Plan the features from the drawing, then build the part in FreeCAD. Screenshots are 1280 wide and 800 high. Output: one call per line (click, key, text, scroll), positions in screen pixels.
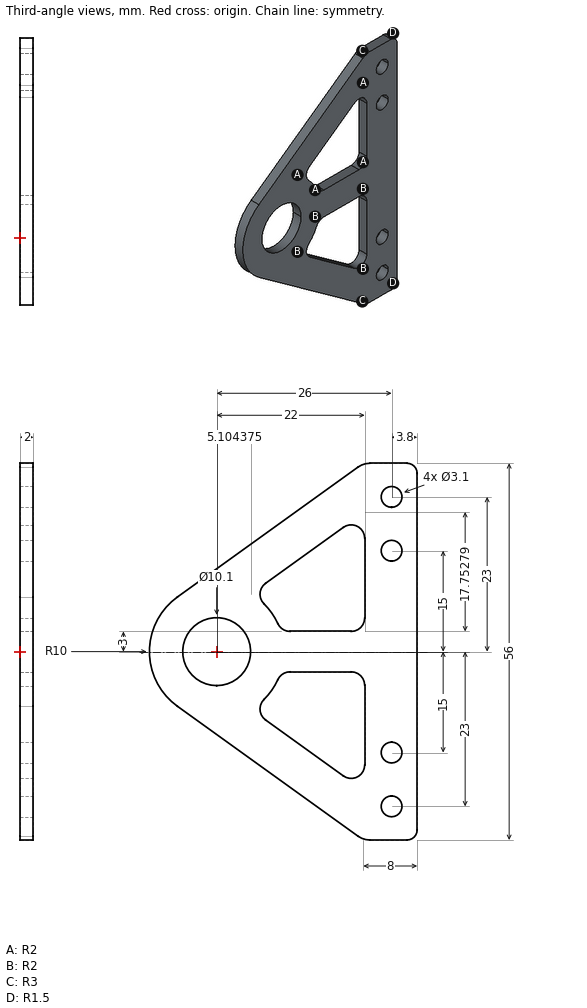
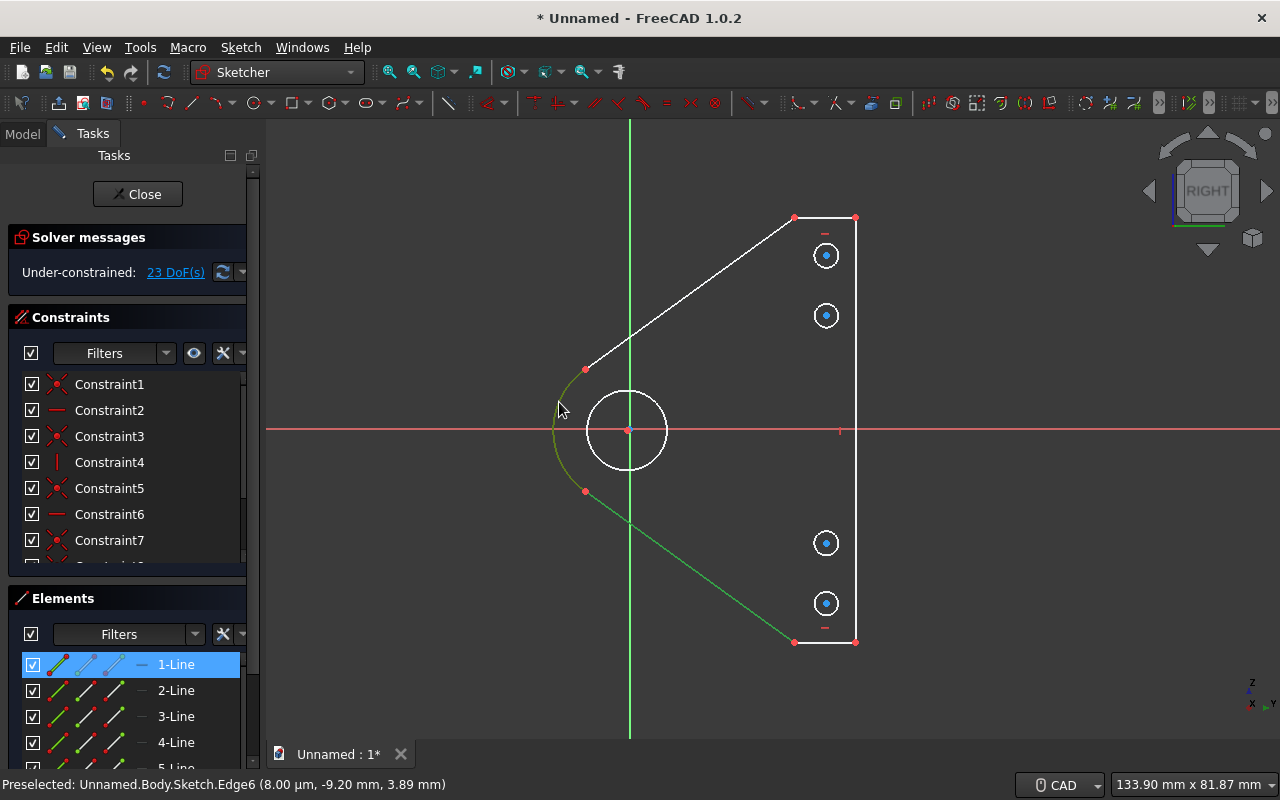
click(644, 104)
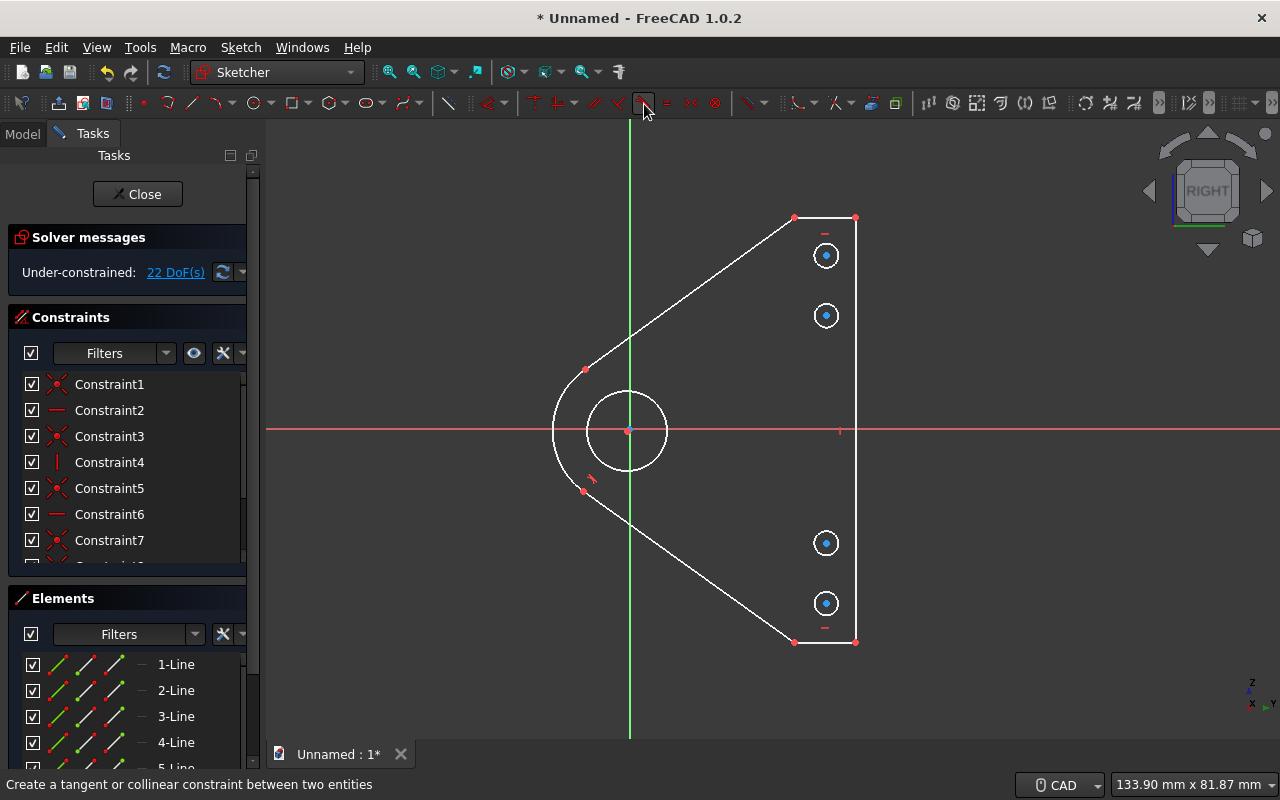
click(732, 263)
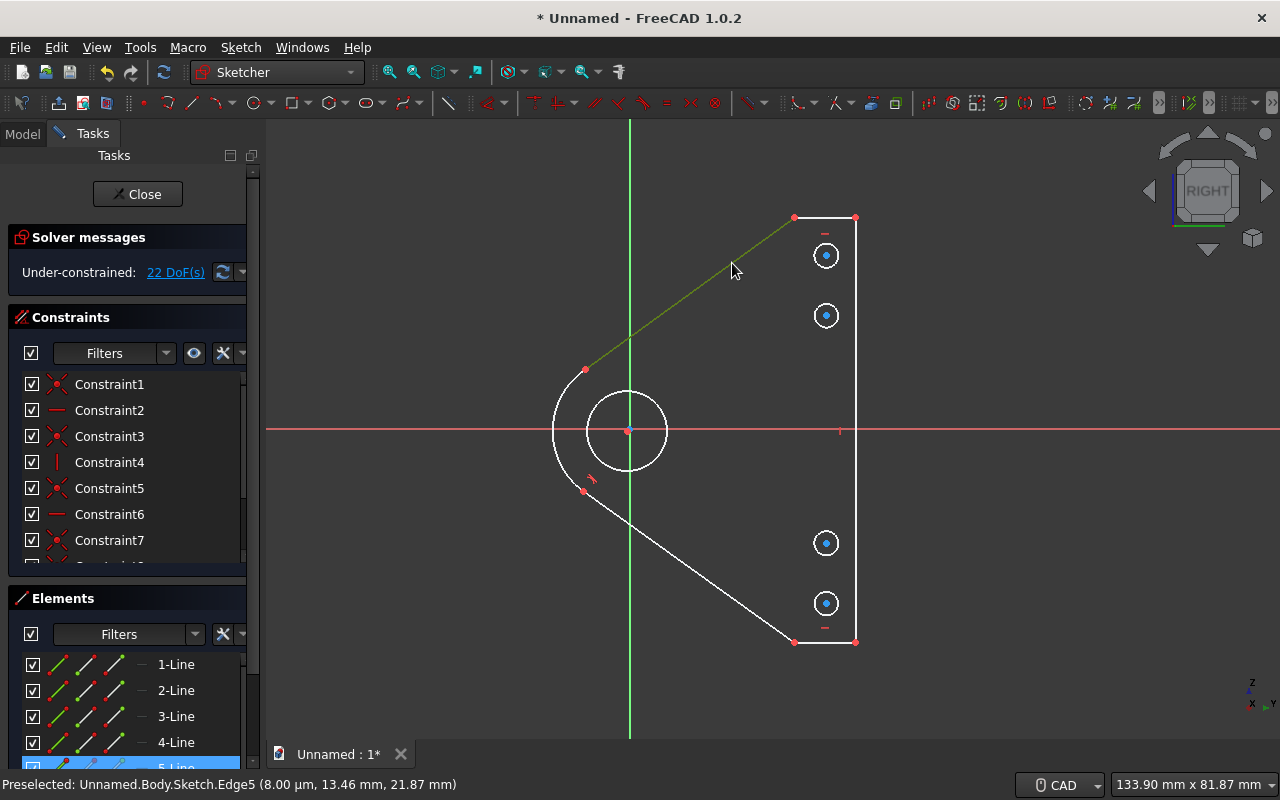
click(559, 402)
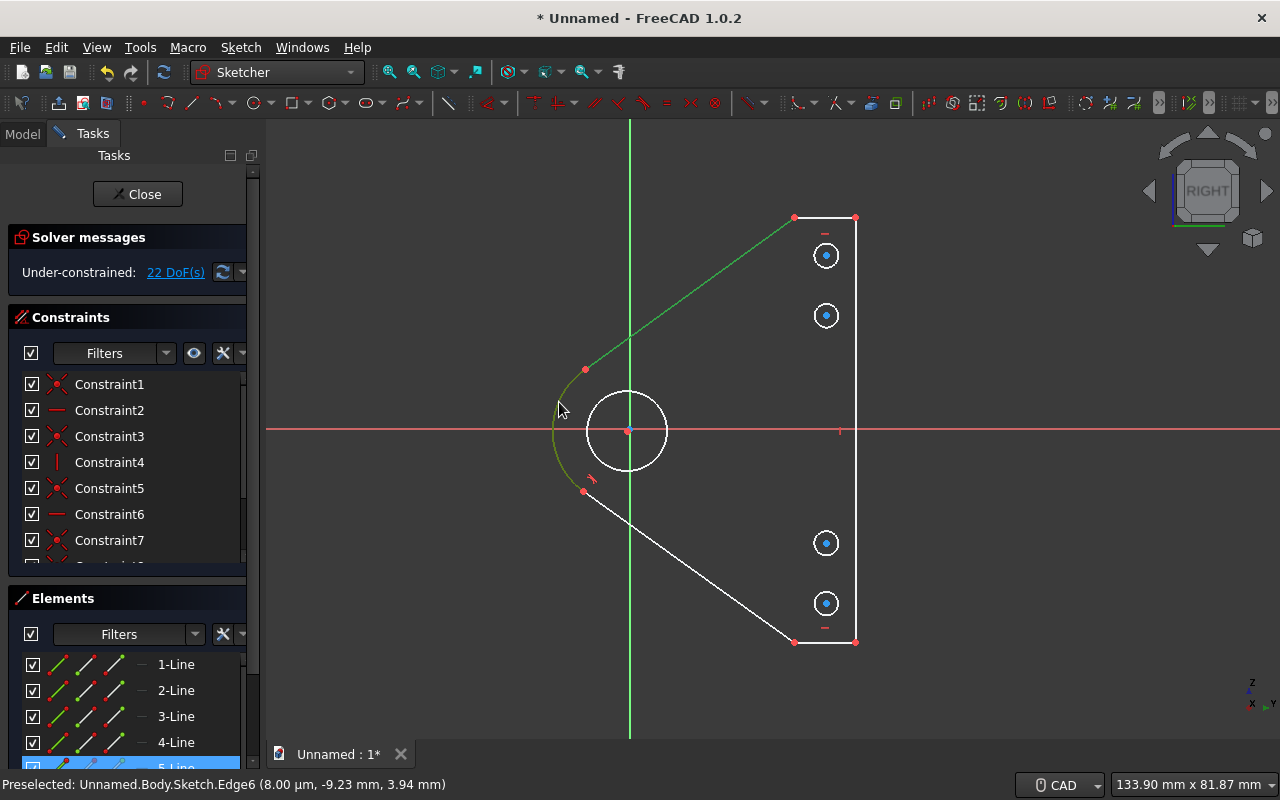
click(644, 104)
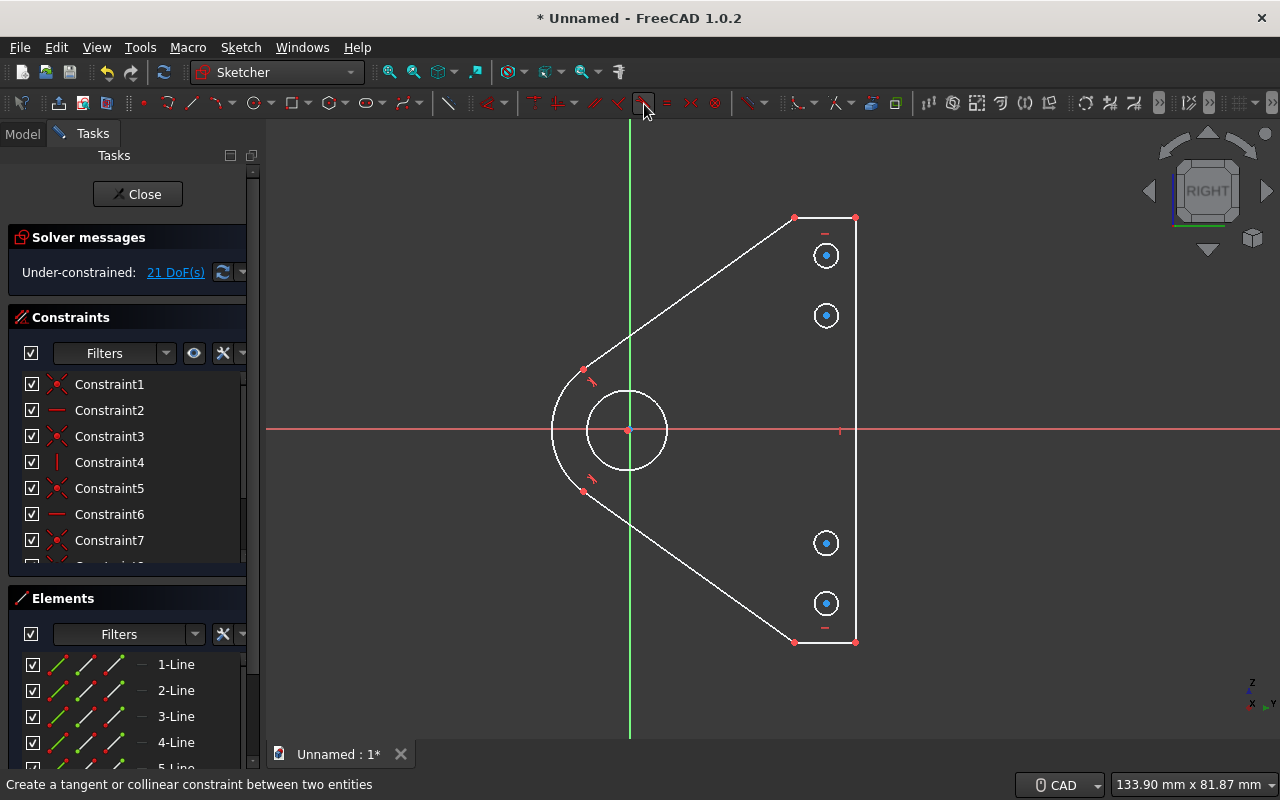
scroll(628, 430, up, 7)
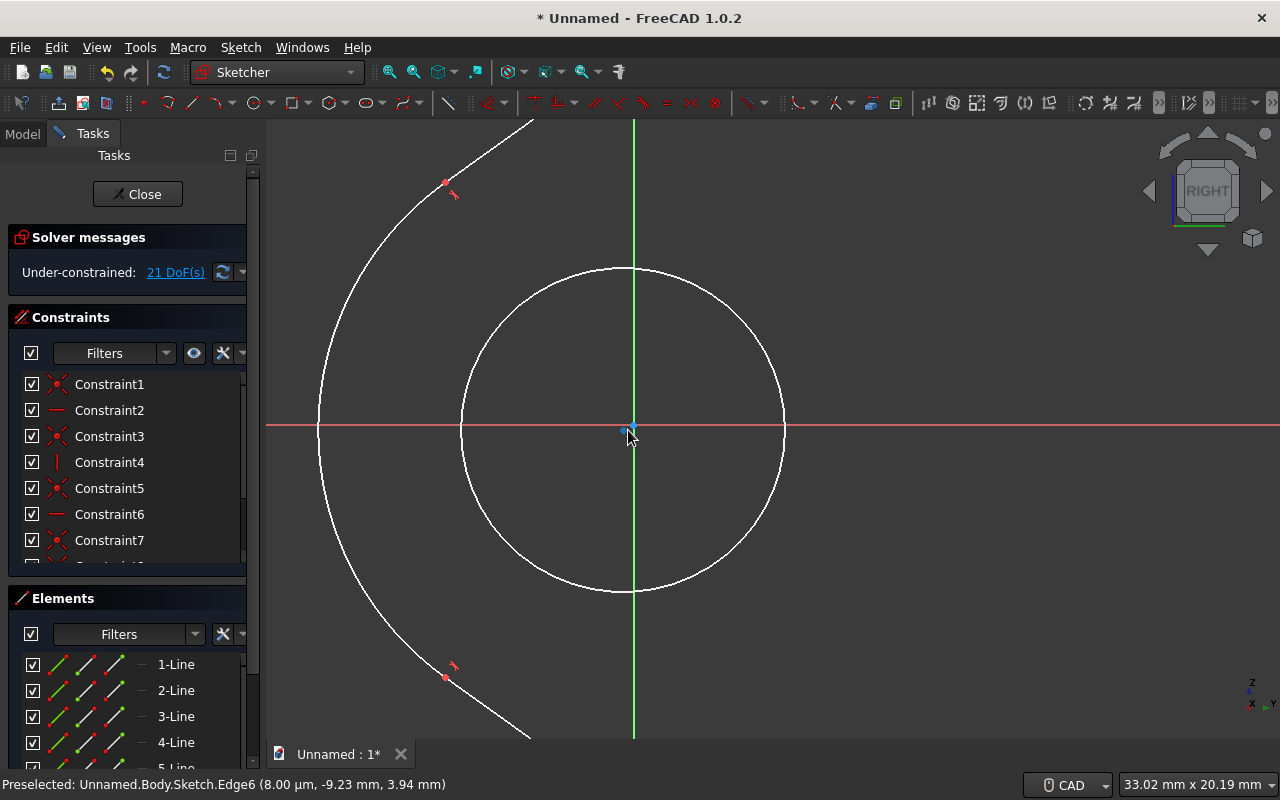
drag(613, 415, 644, 440)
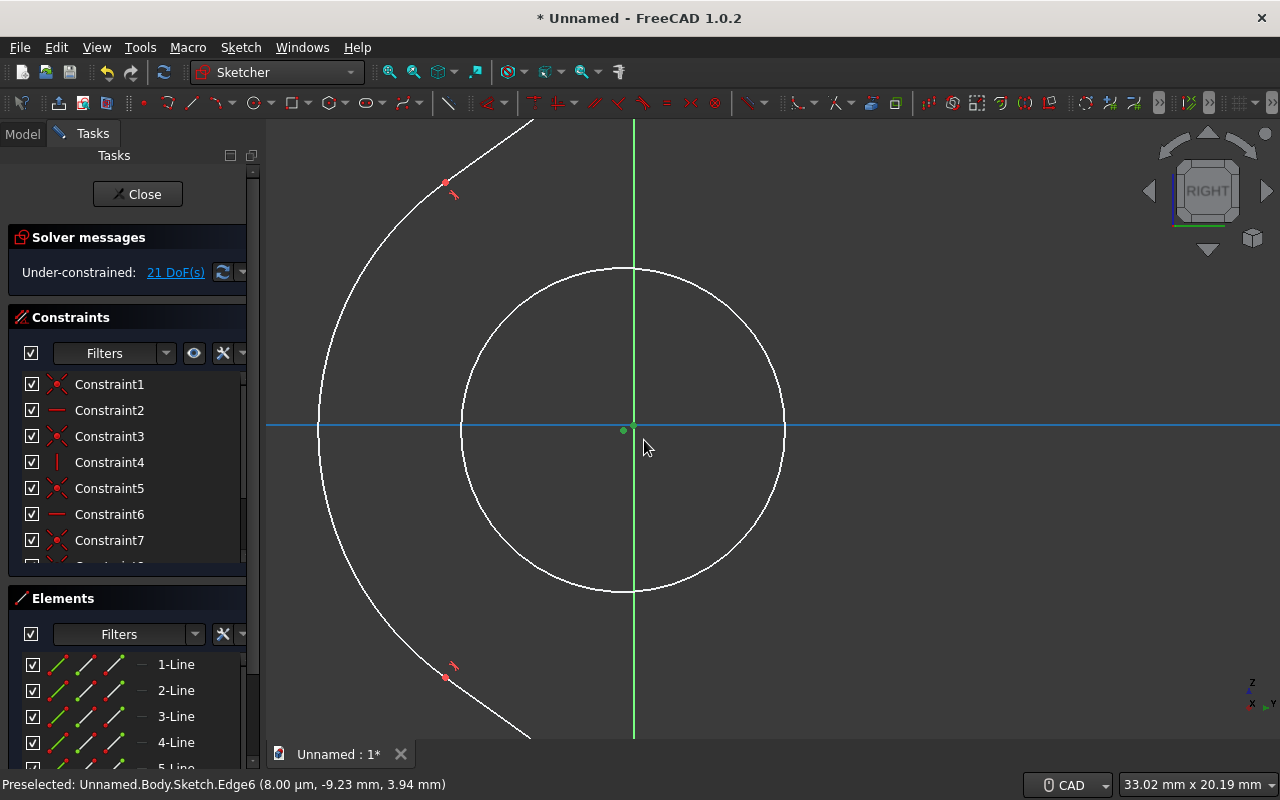
click(534, 104)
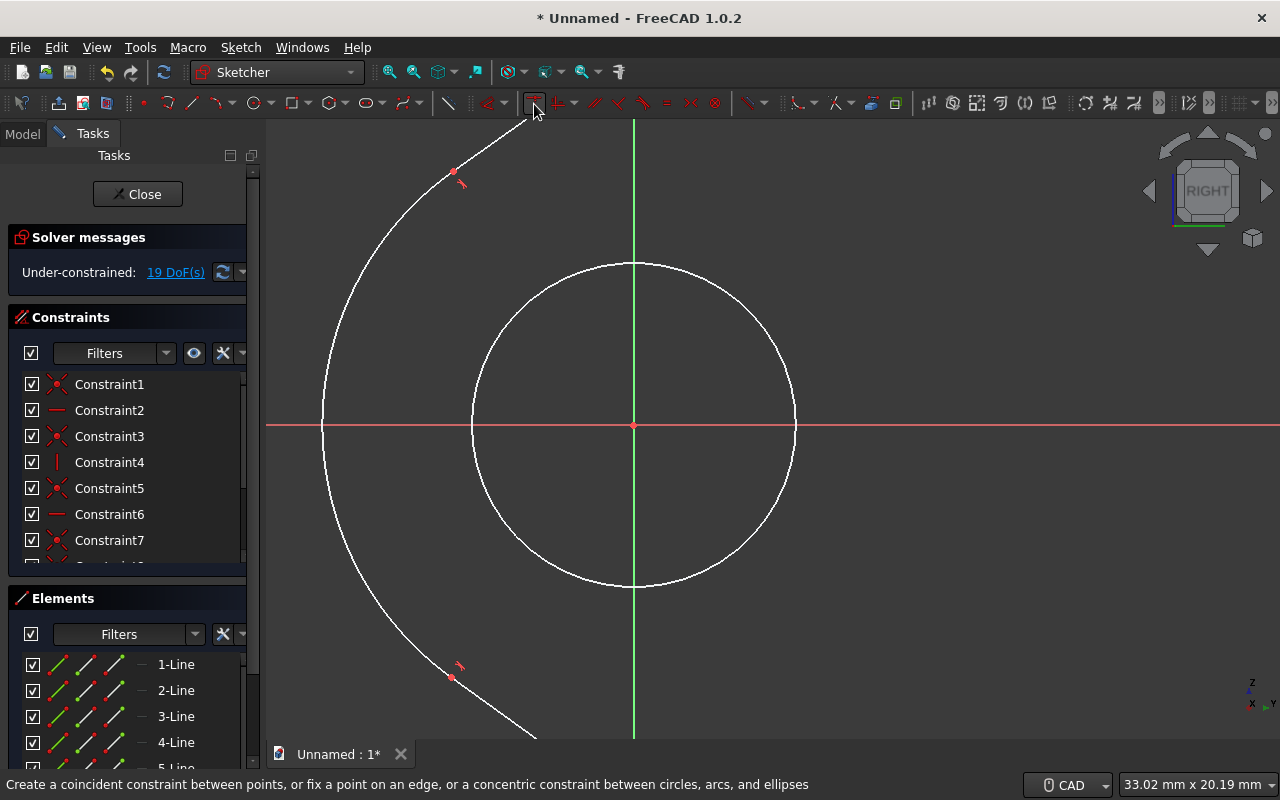
scroll(628, 430, down, 7)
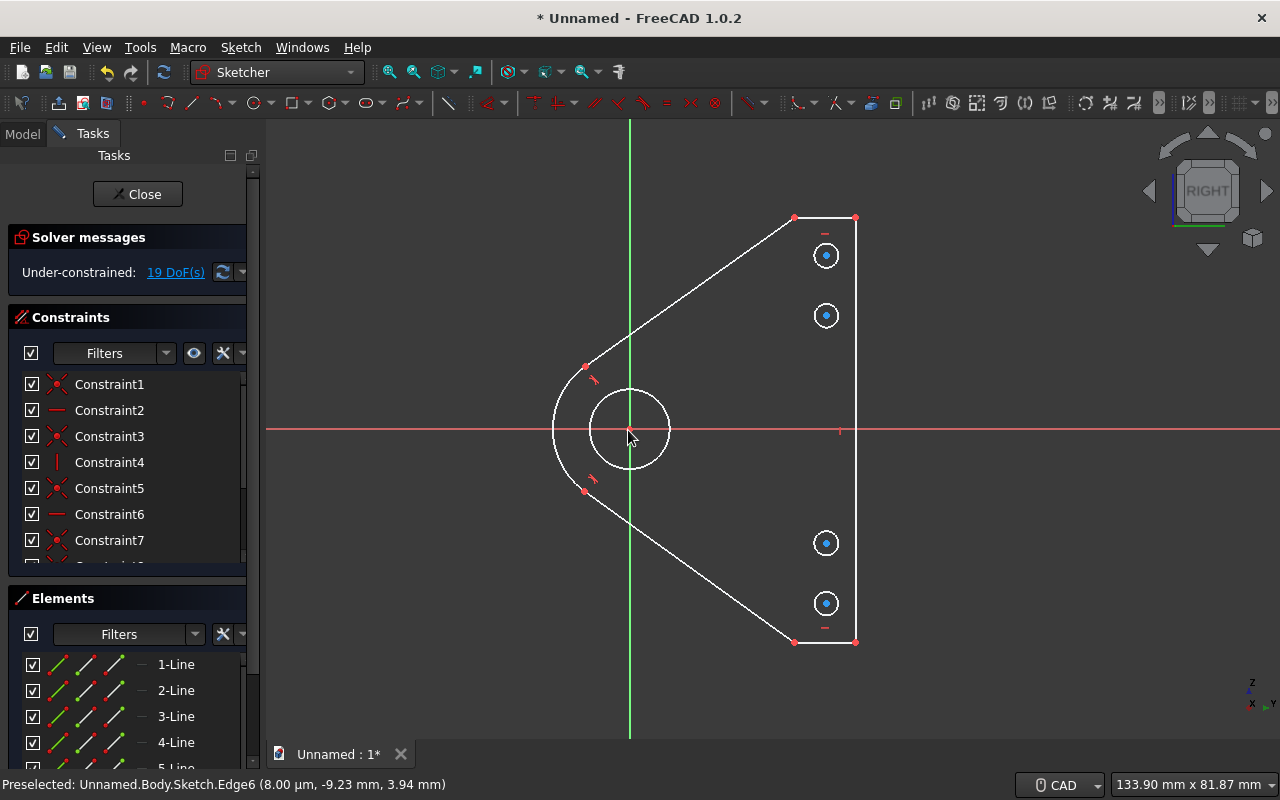
click(835, 247)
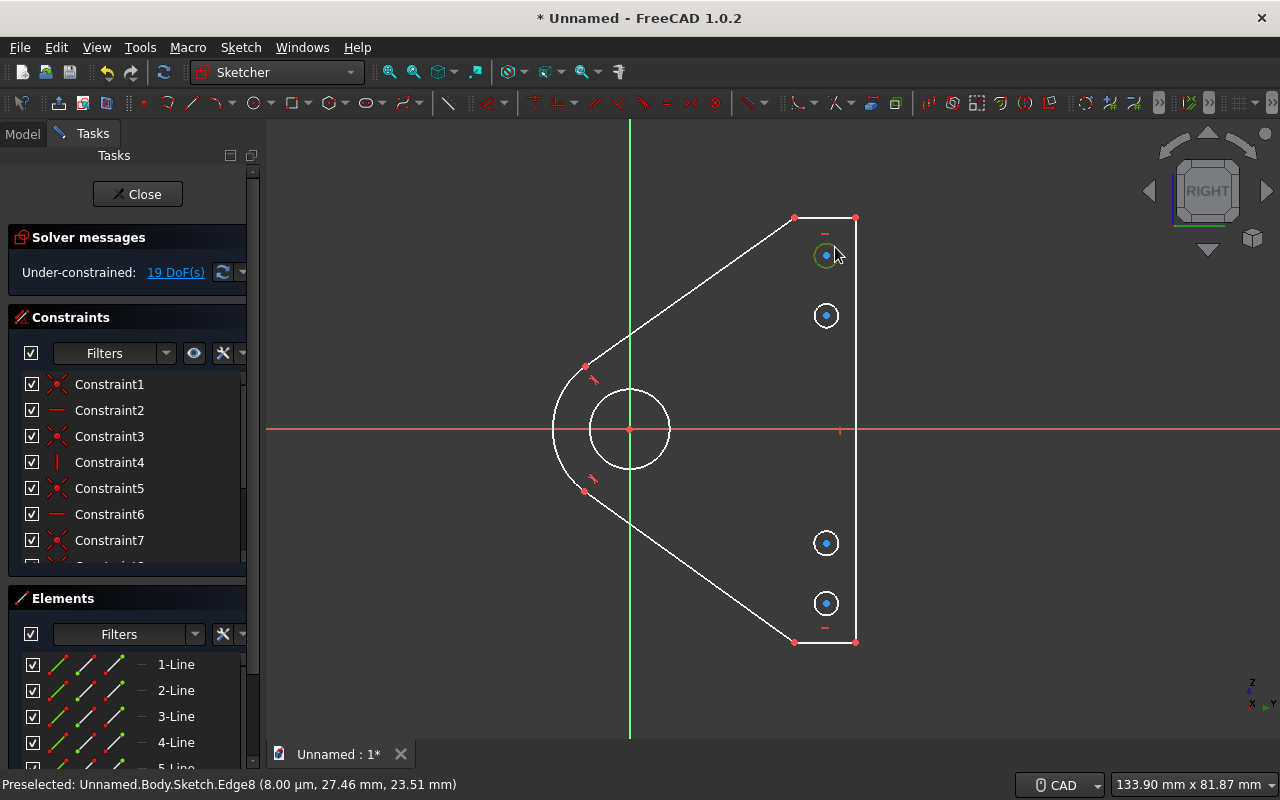
click(835, 307)